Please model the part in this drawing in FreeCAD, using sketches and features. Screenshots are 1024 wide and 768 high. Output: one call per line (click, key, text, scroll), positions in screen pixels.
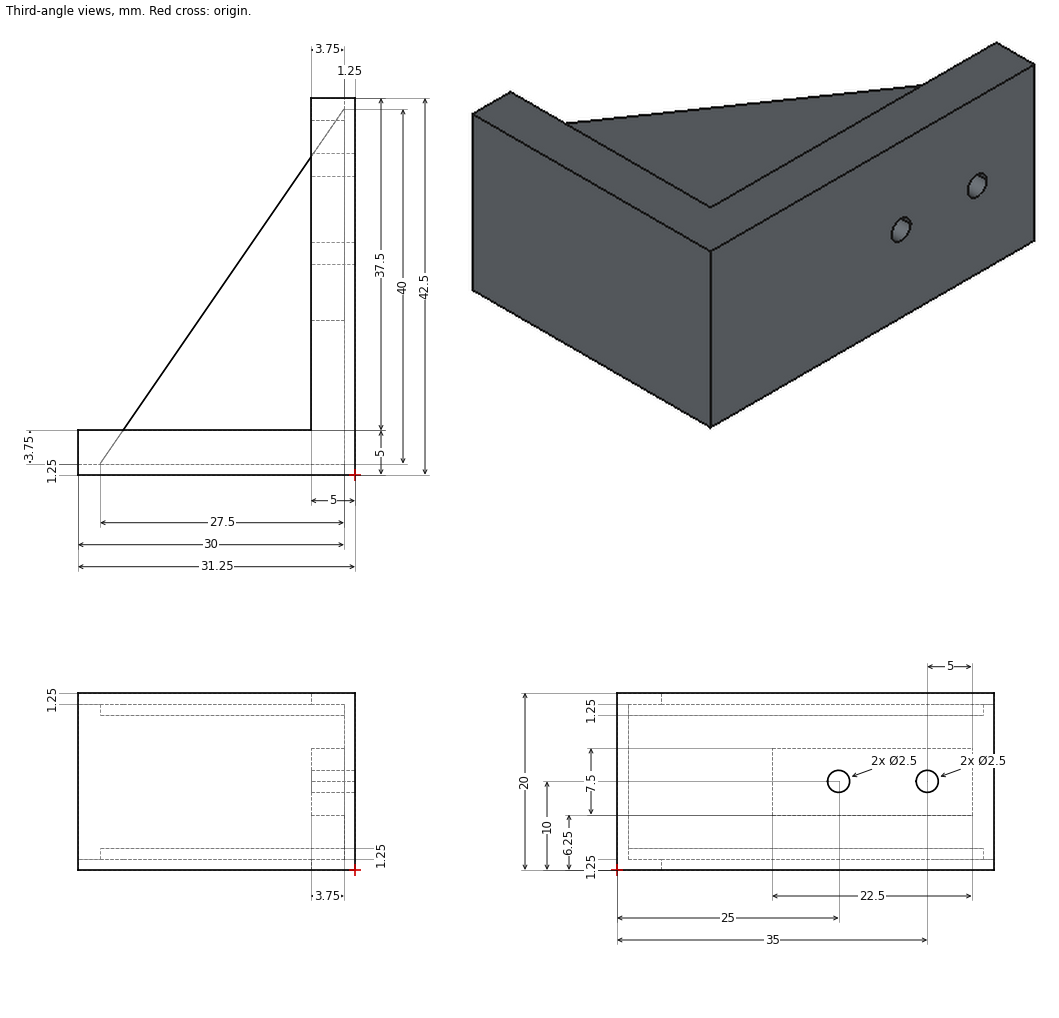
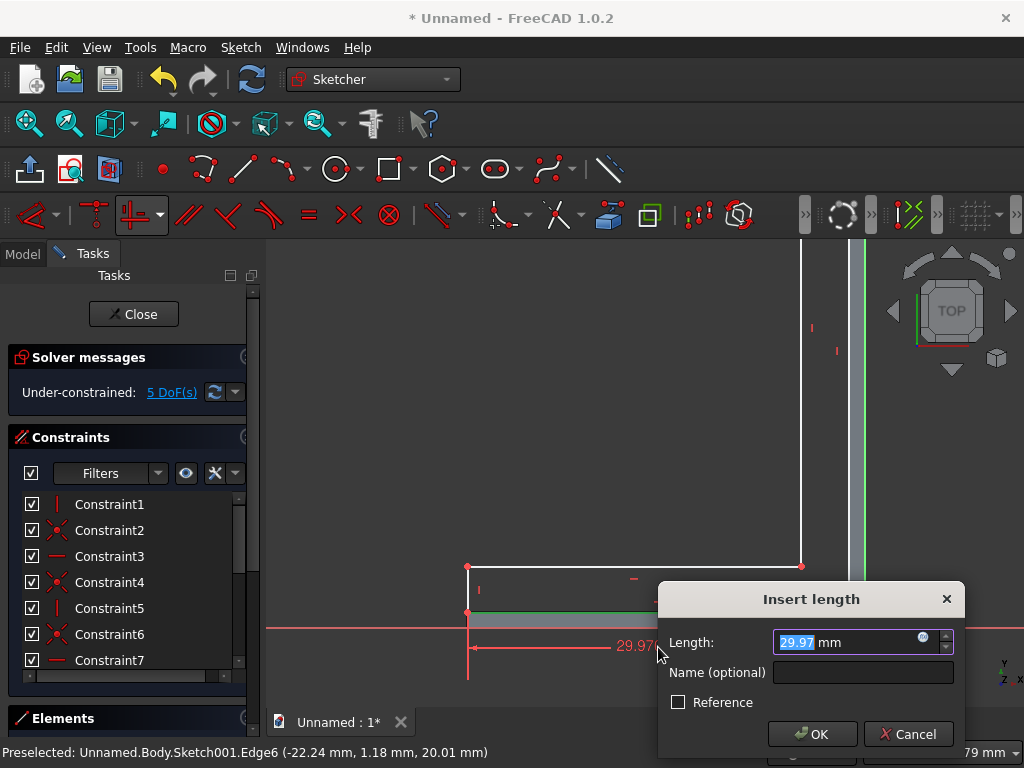
text(30)
key(Return)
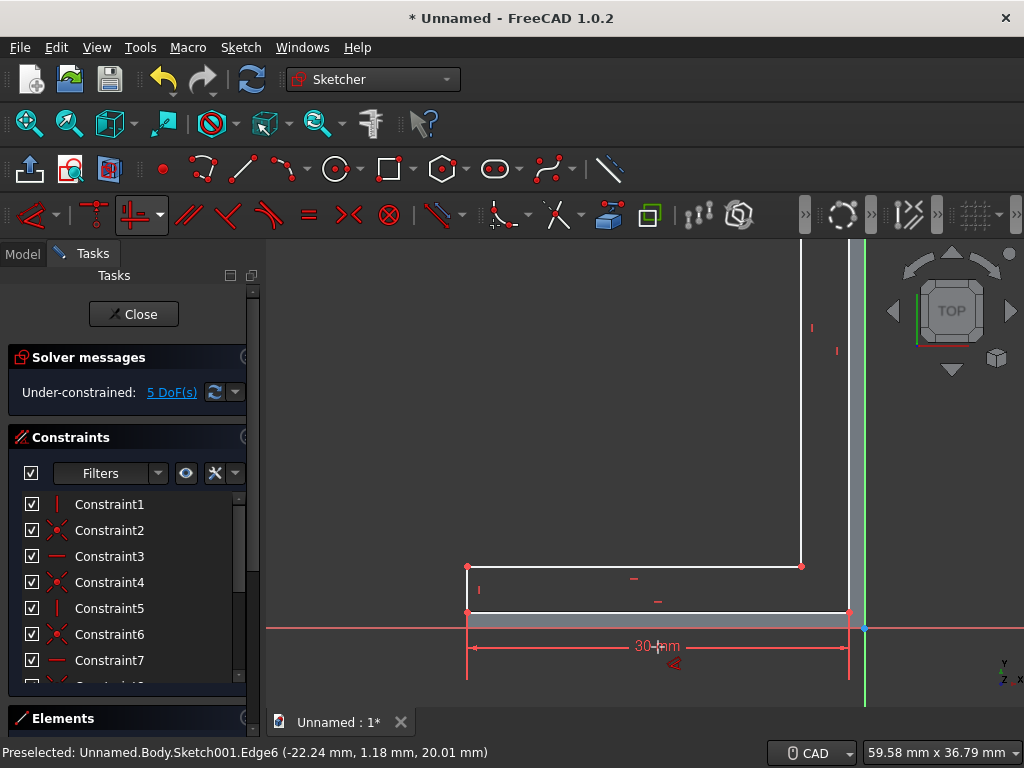
scroll(468, 613, down, 3)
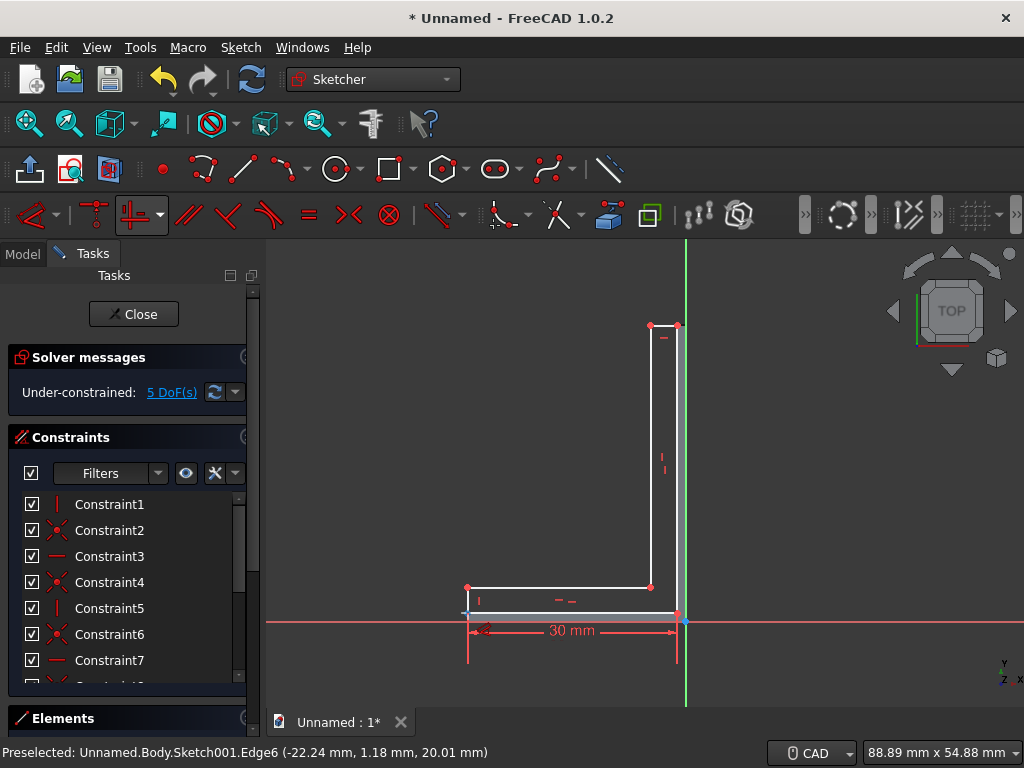
click(651, 326)
click(668, 656)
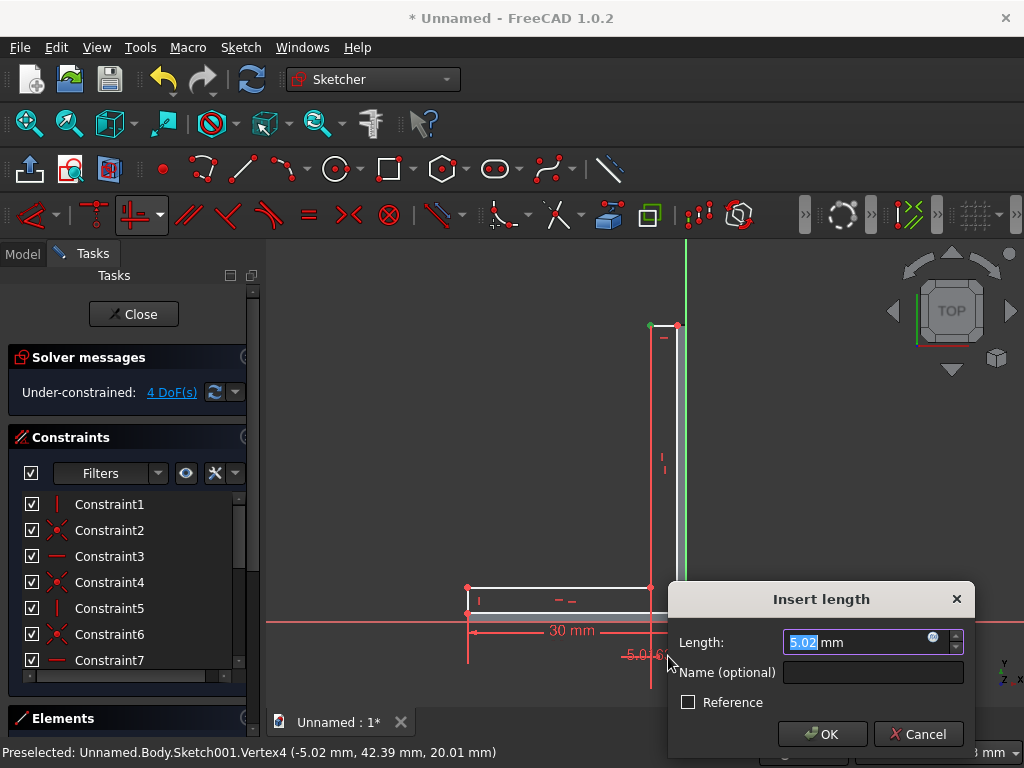
text(5)
key(Return)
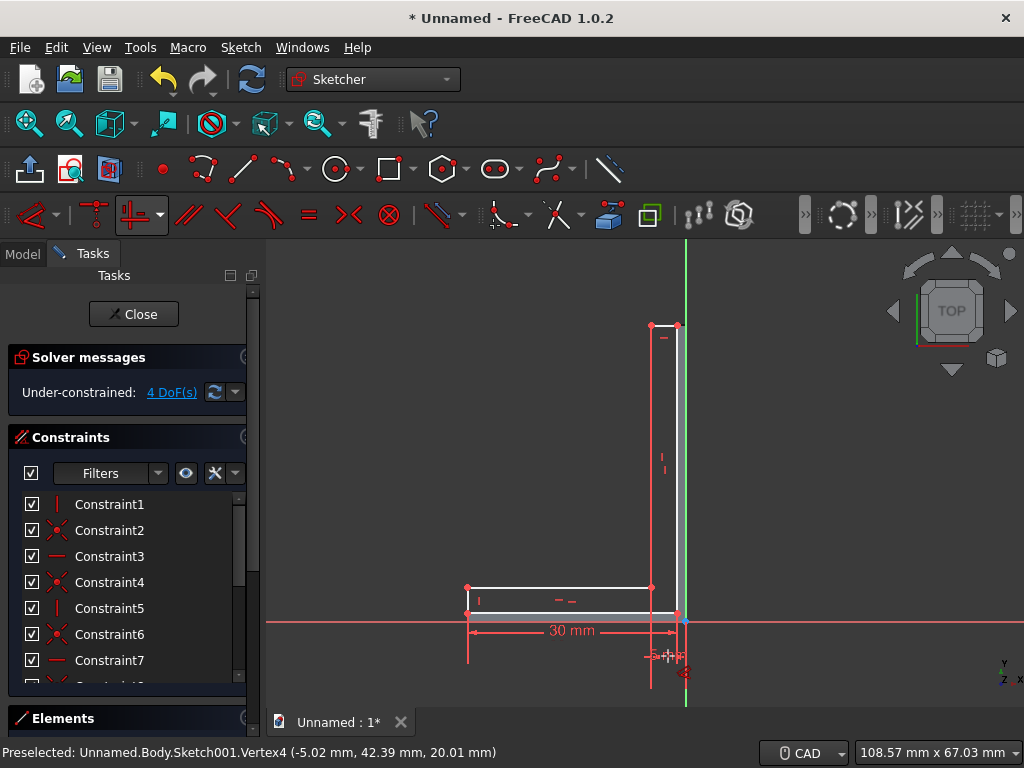
click(651, 588)
click(720, 605)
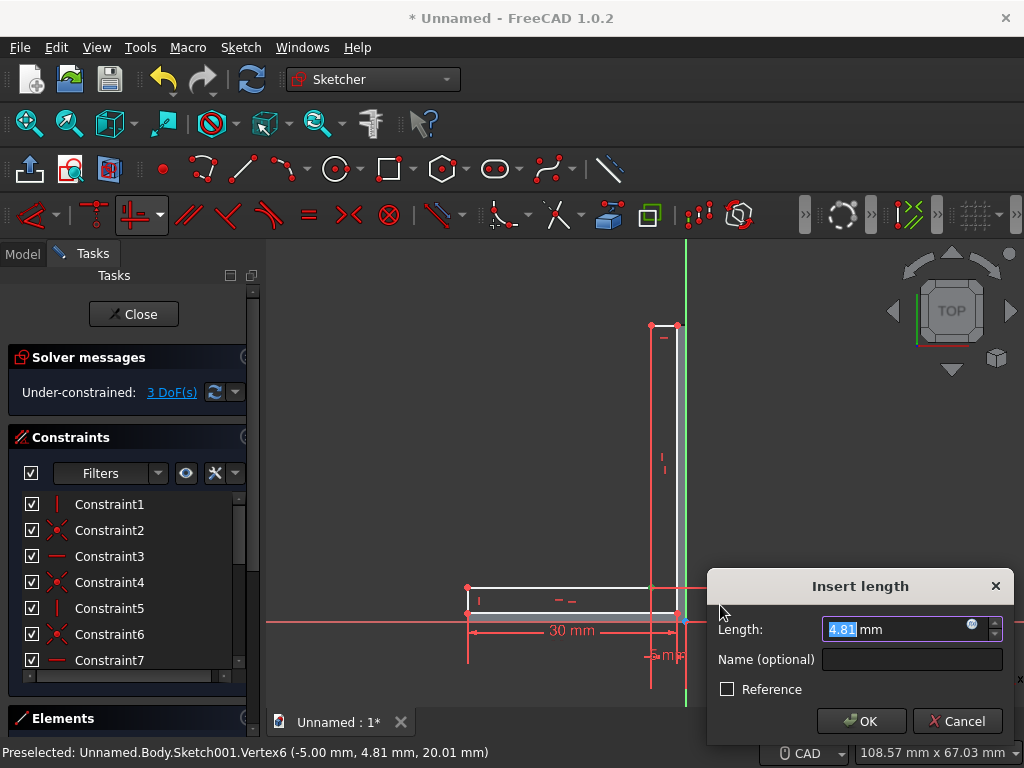
text(5)
key(Return)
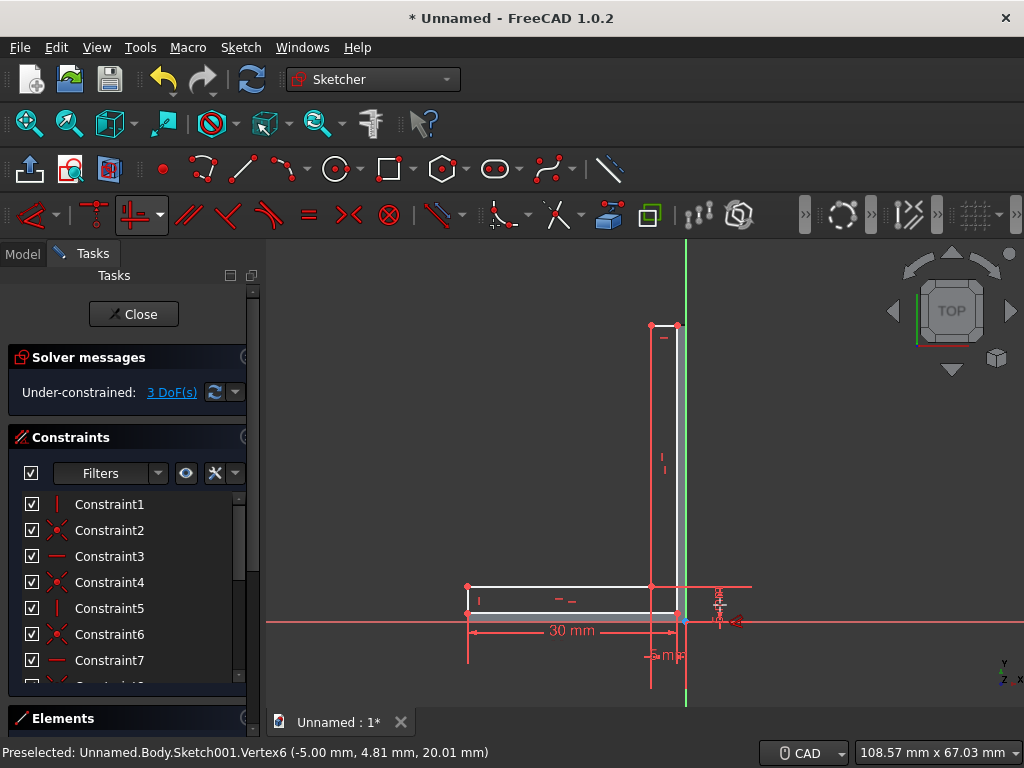
scroll(667, 326, up, 3)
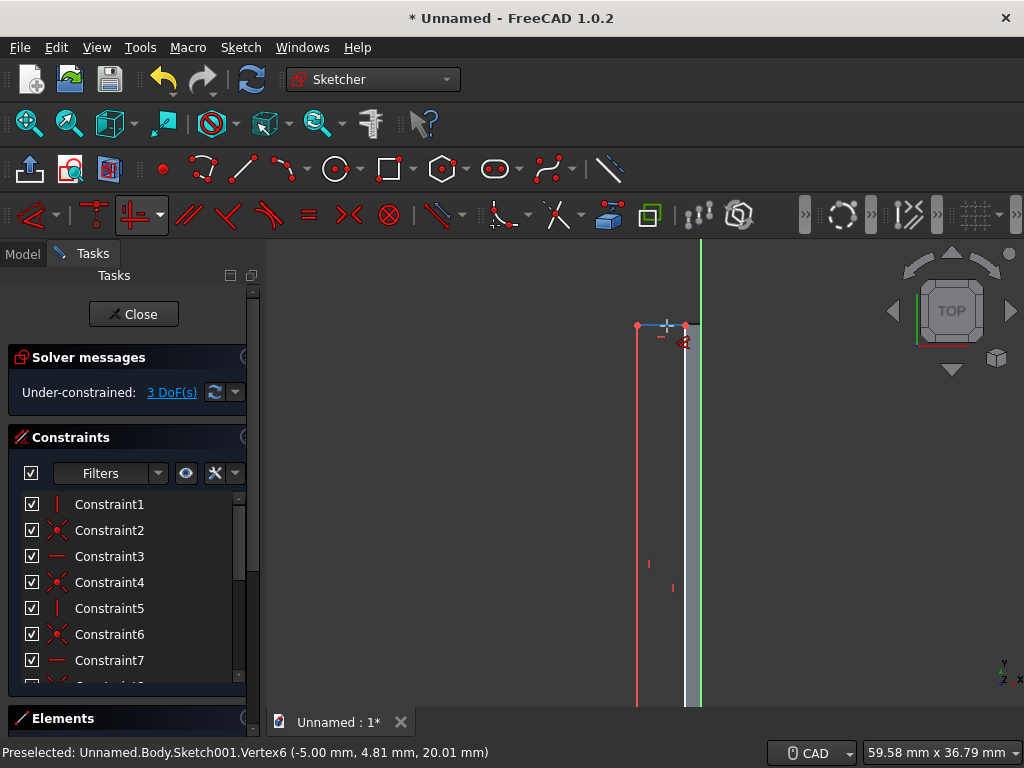
click(666, 325)
click(661, 291)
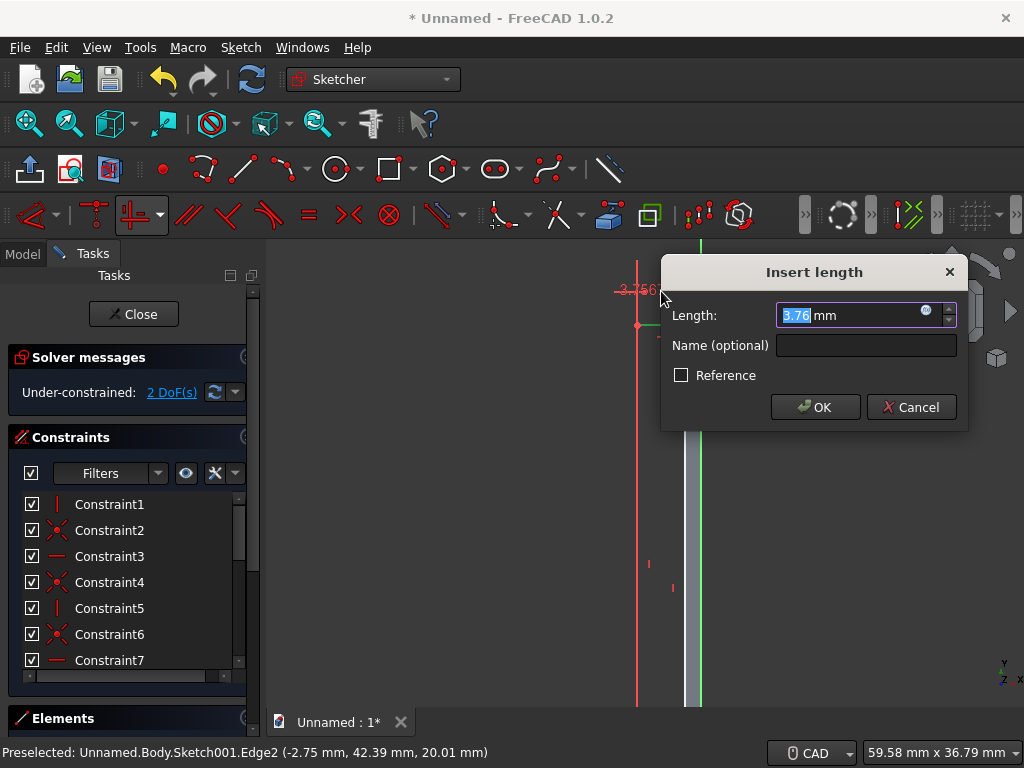
text(3.75)
key(Return)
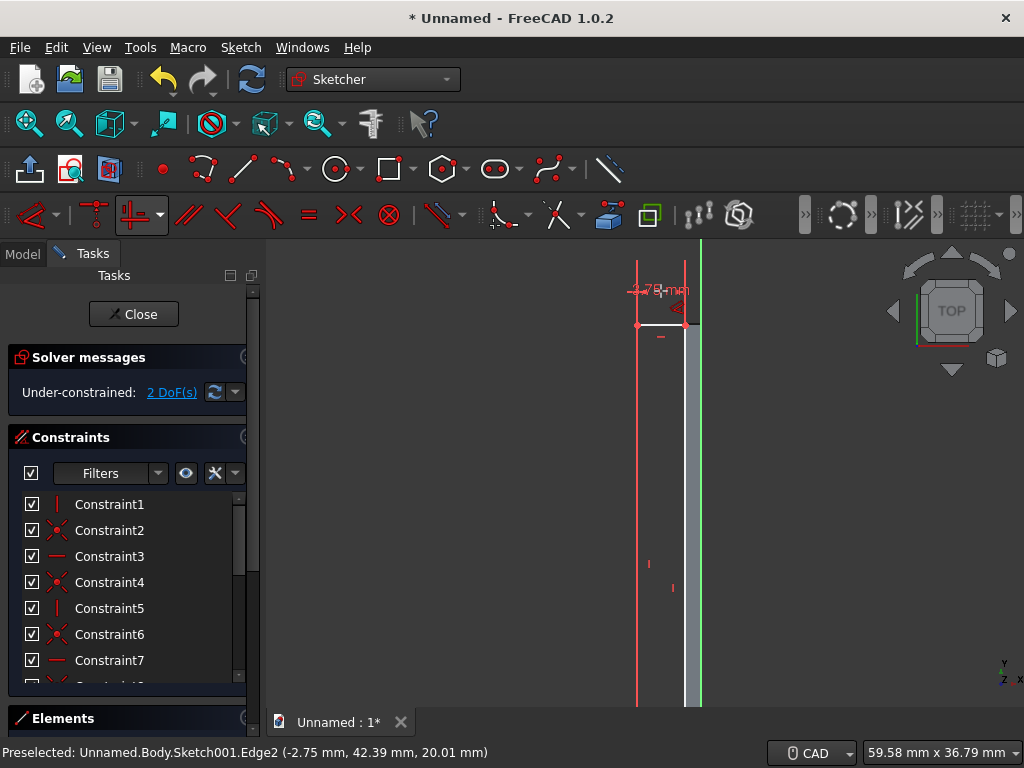
click(637, 468)
click(671, 502)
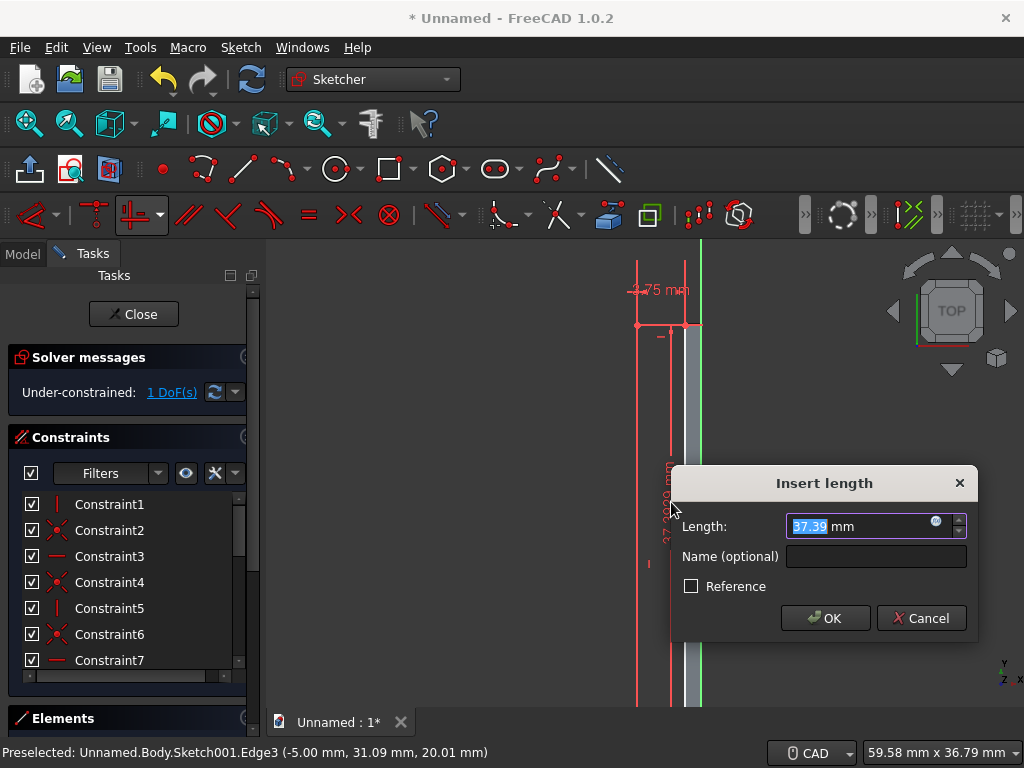
text(37.5)
key(Return)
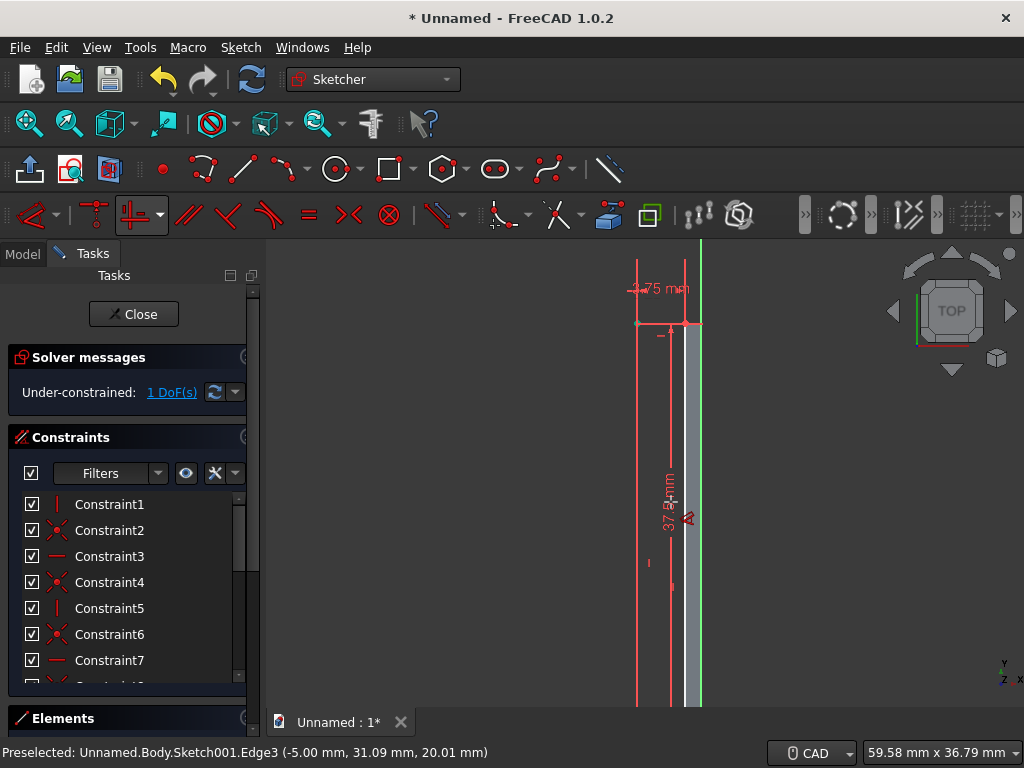
scroll(667, 326, down, 3)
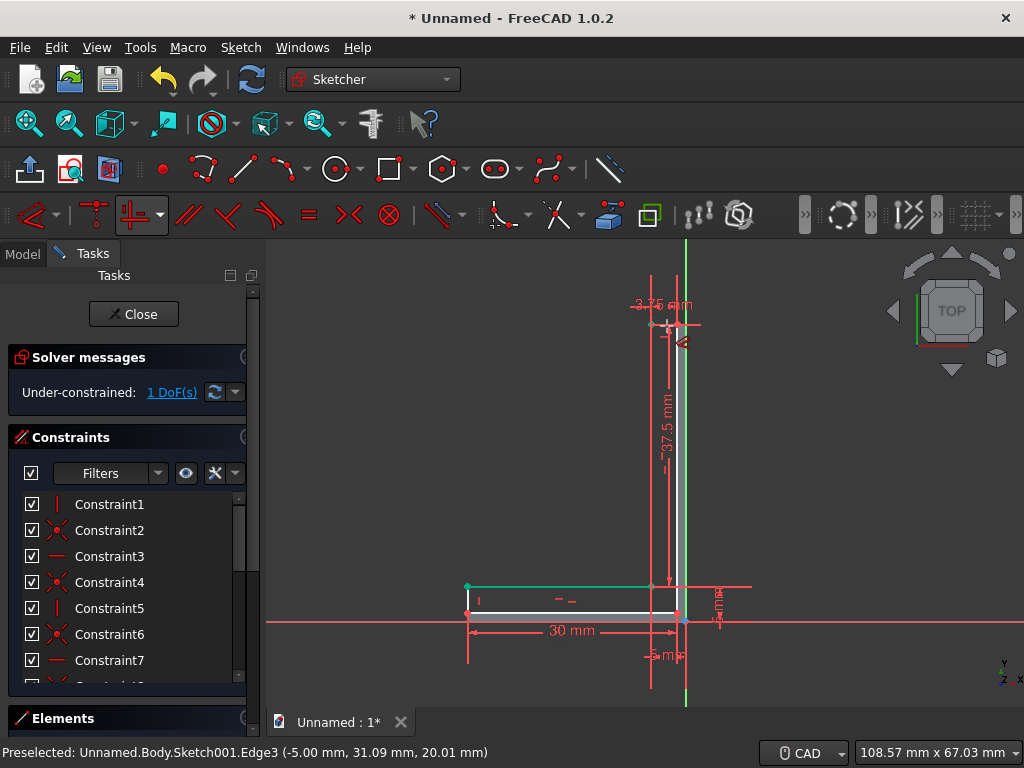
scroll(468, 595, up, 3)